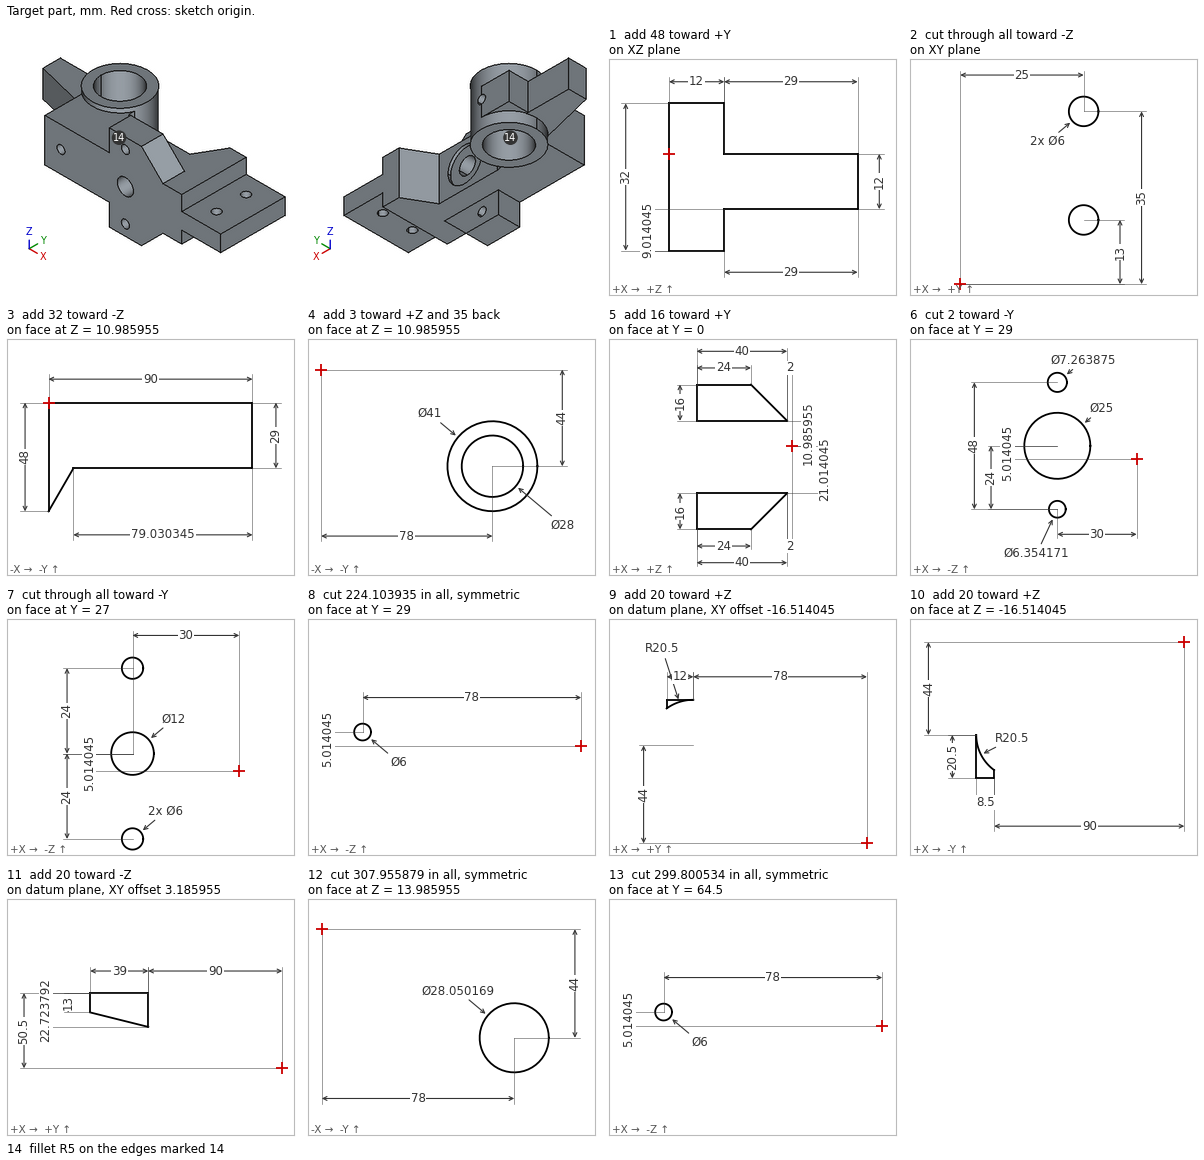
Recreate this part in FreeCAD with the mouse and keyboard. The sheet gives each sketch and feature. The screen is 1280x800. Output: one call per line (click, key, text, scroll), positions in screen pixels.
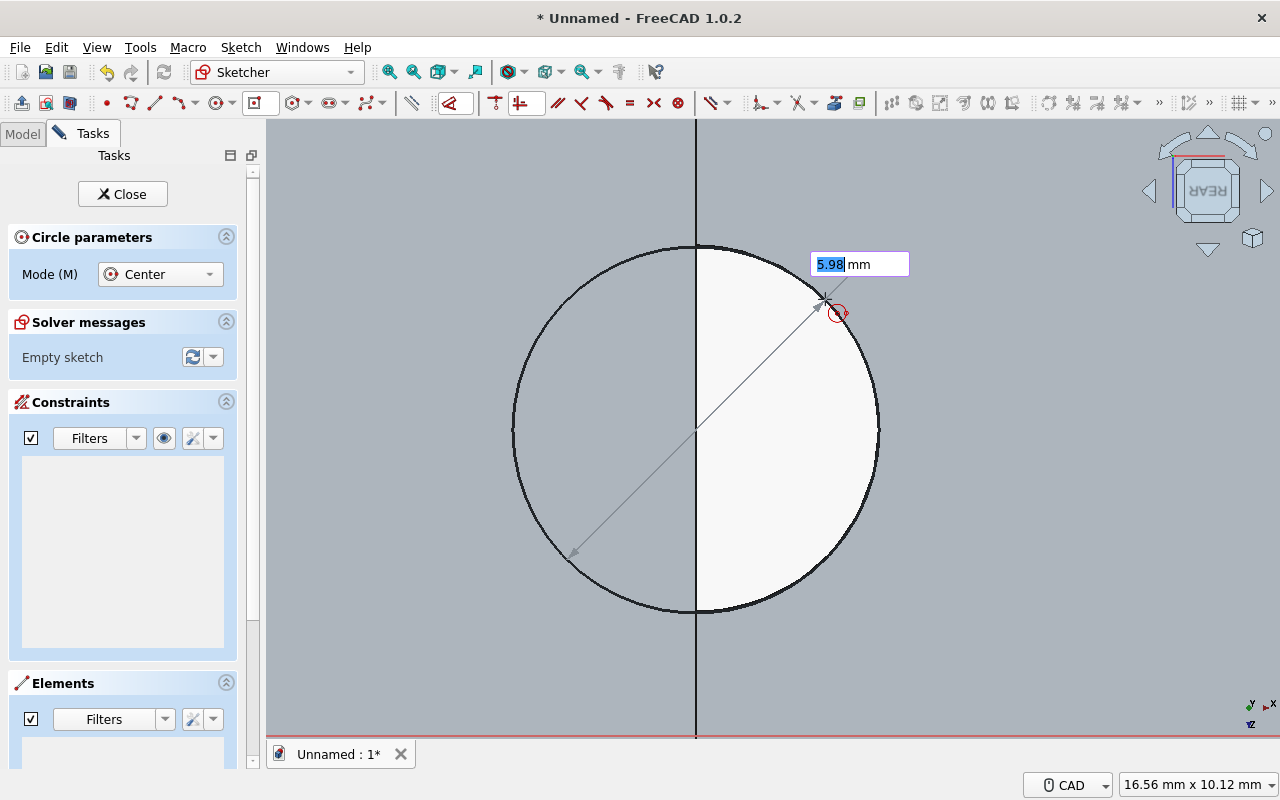
text(6)
key(Return)
key(Escape)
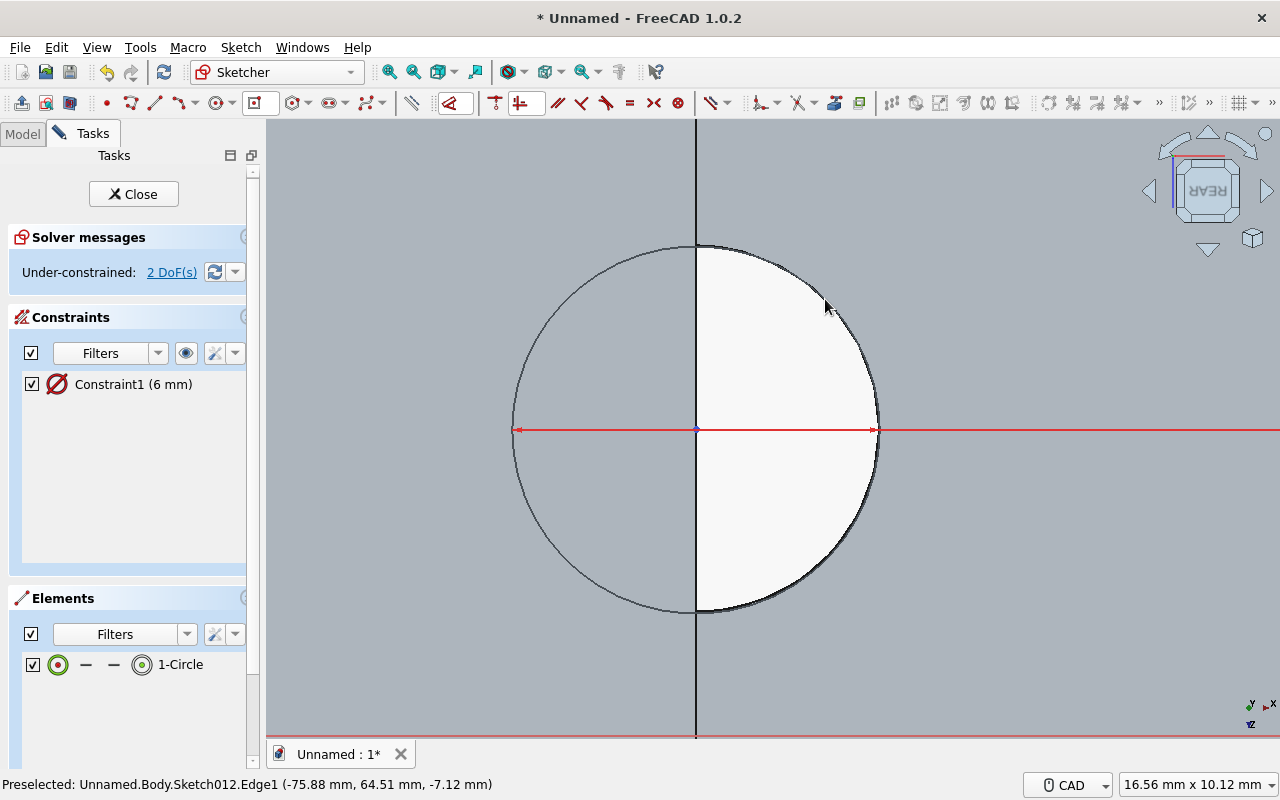
click(696, 430)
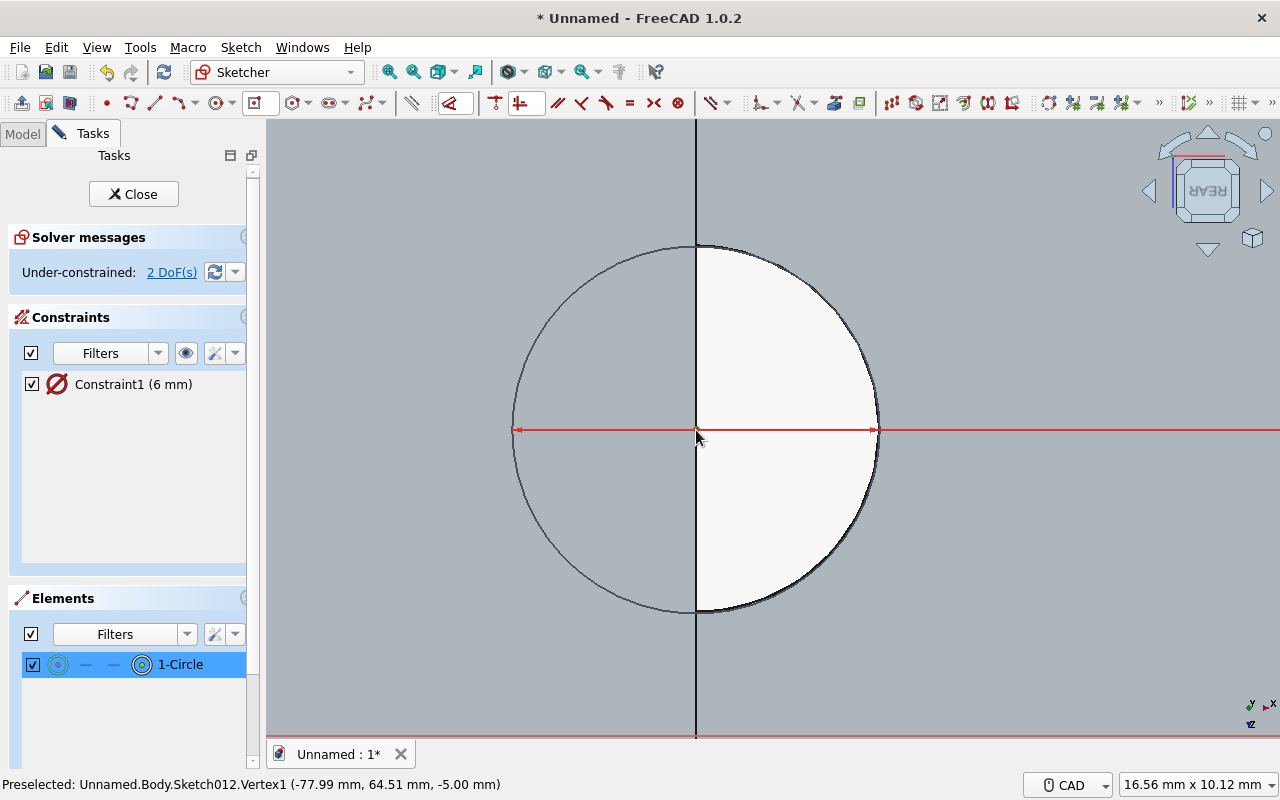
key(l)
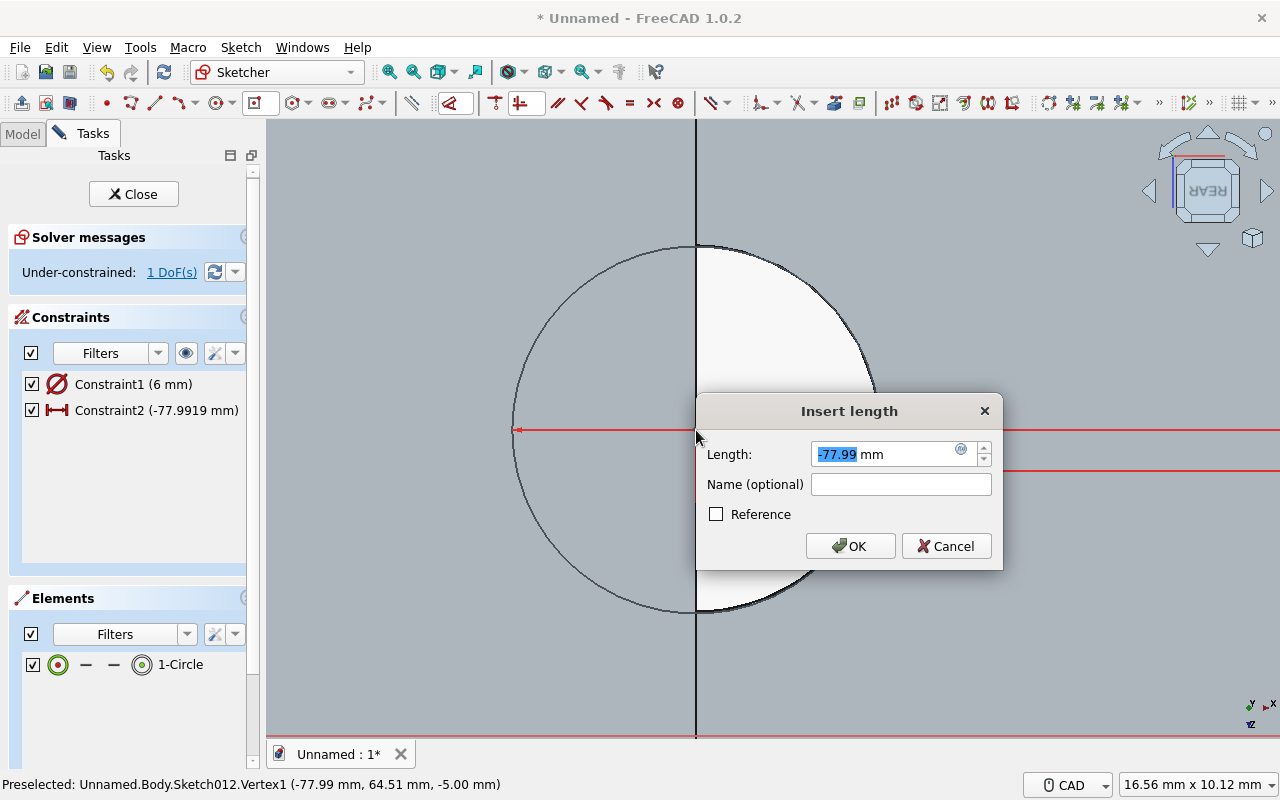
text(-78)
key(Return)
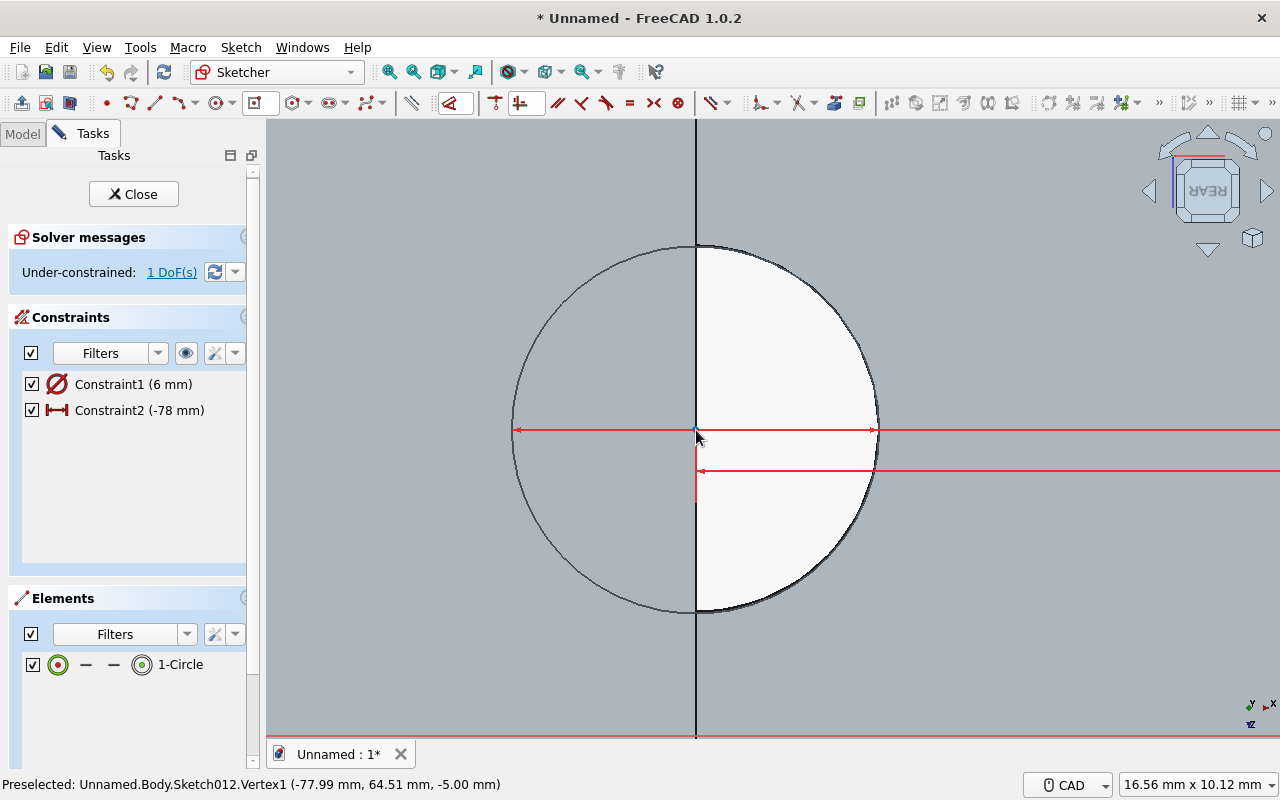
click(696, 430)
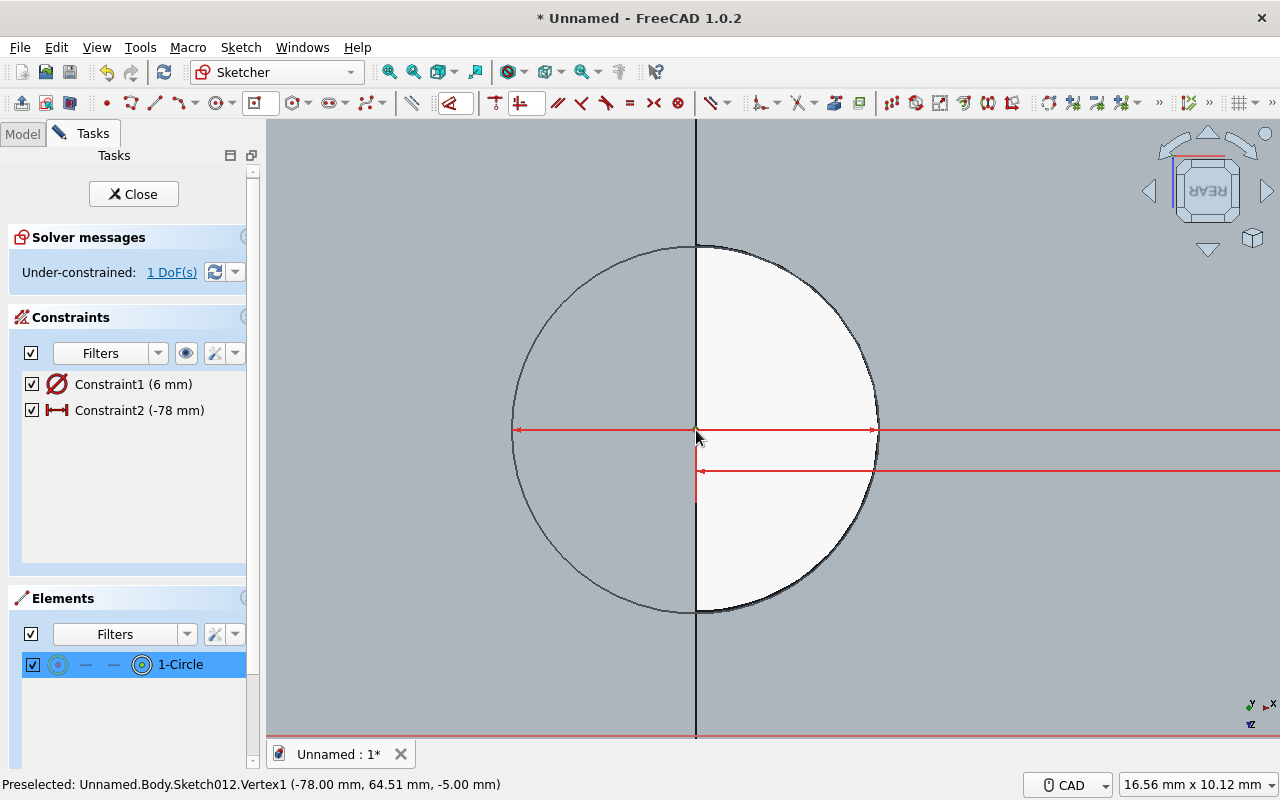
key(i)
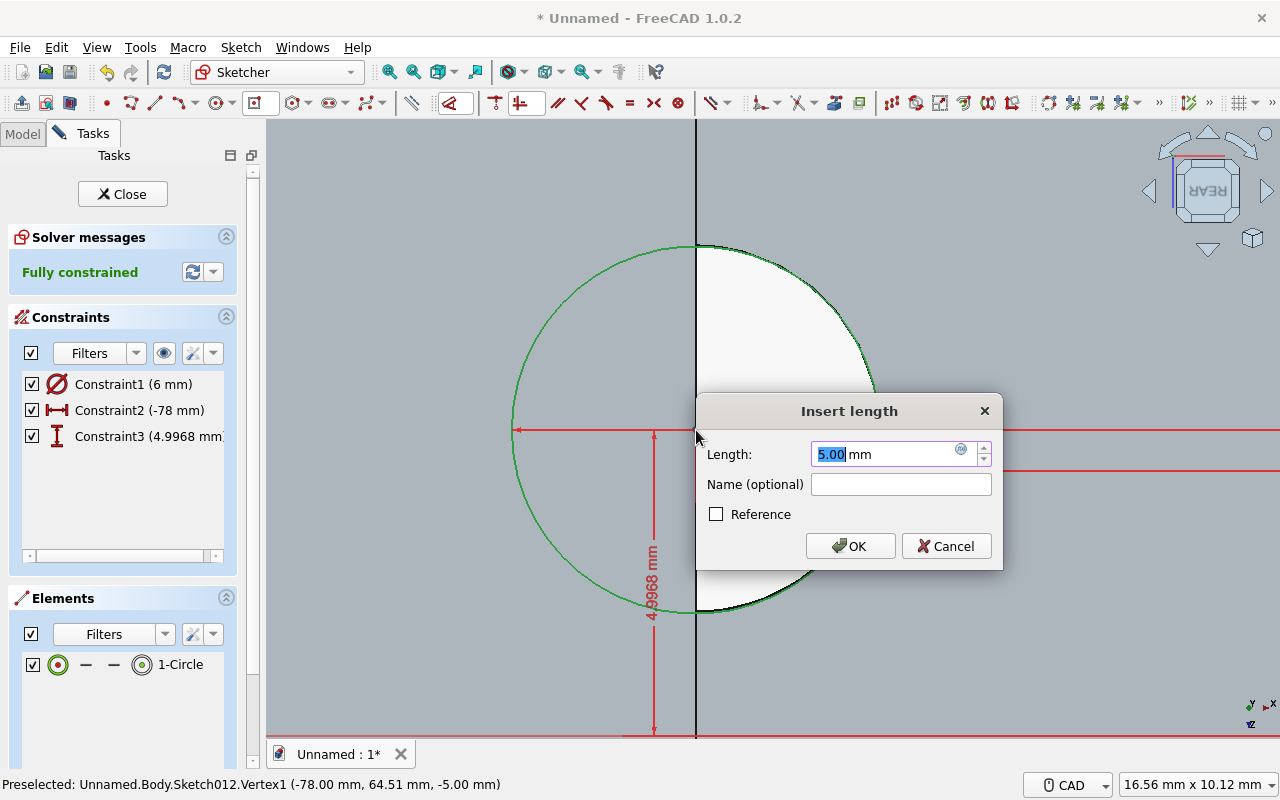
text(5.014045)
key(Return)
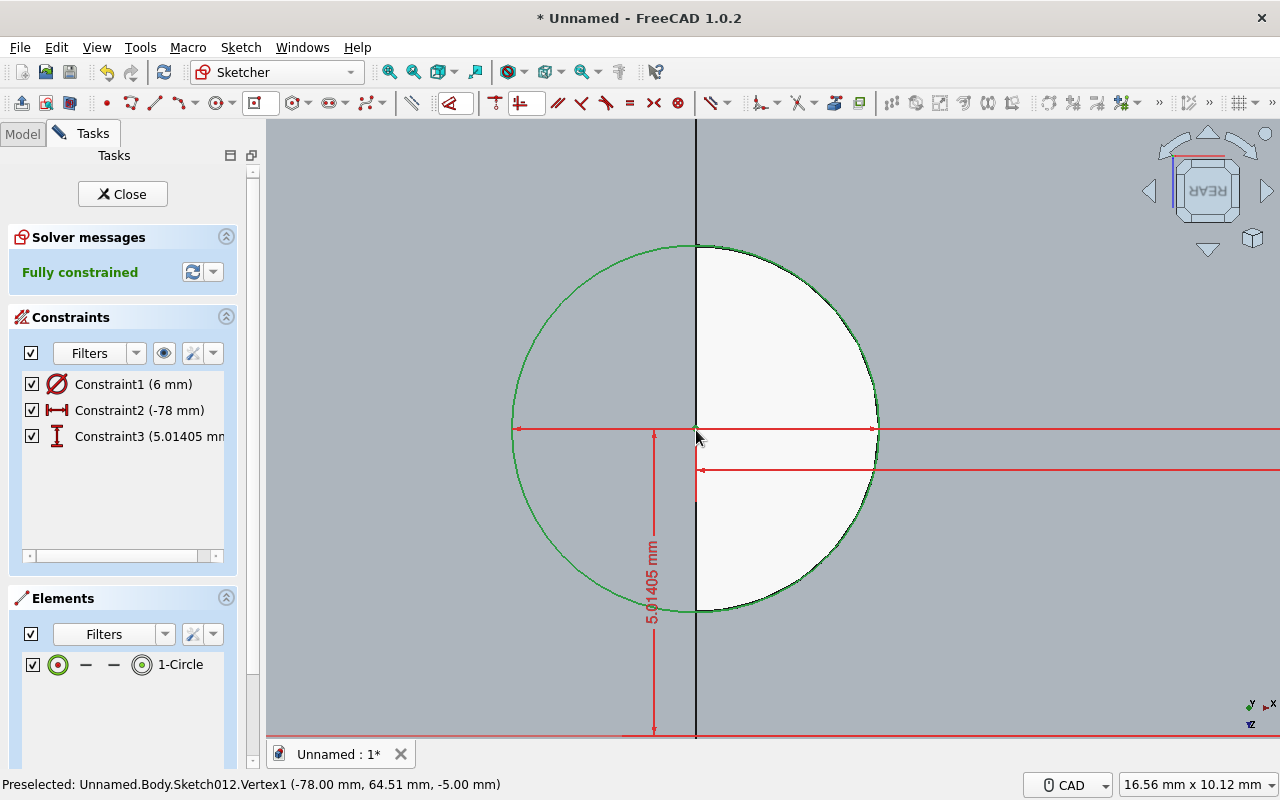
click(123, 194)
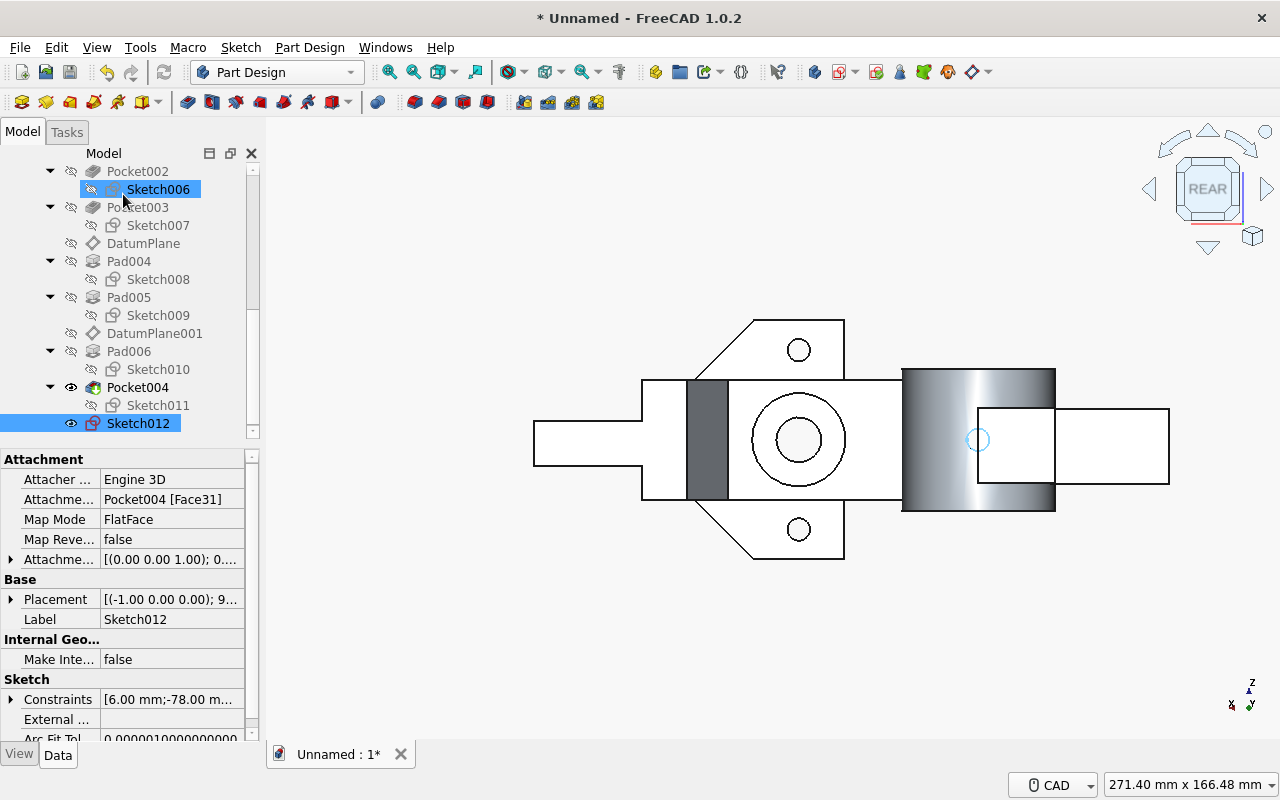
click(188, 102)